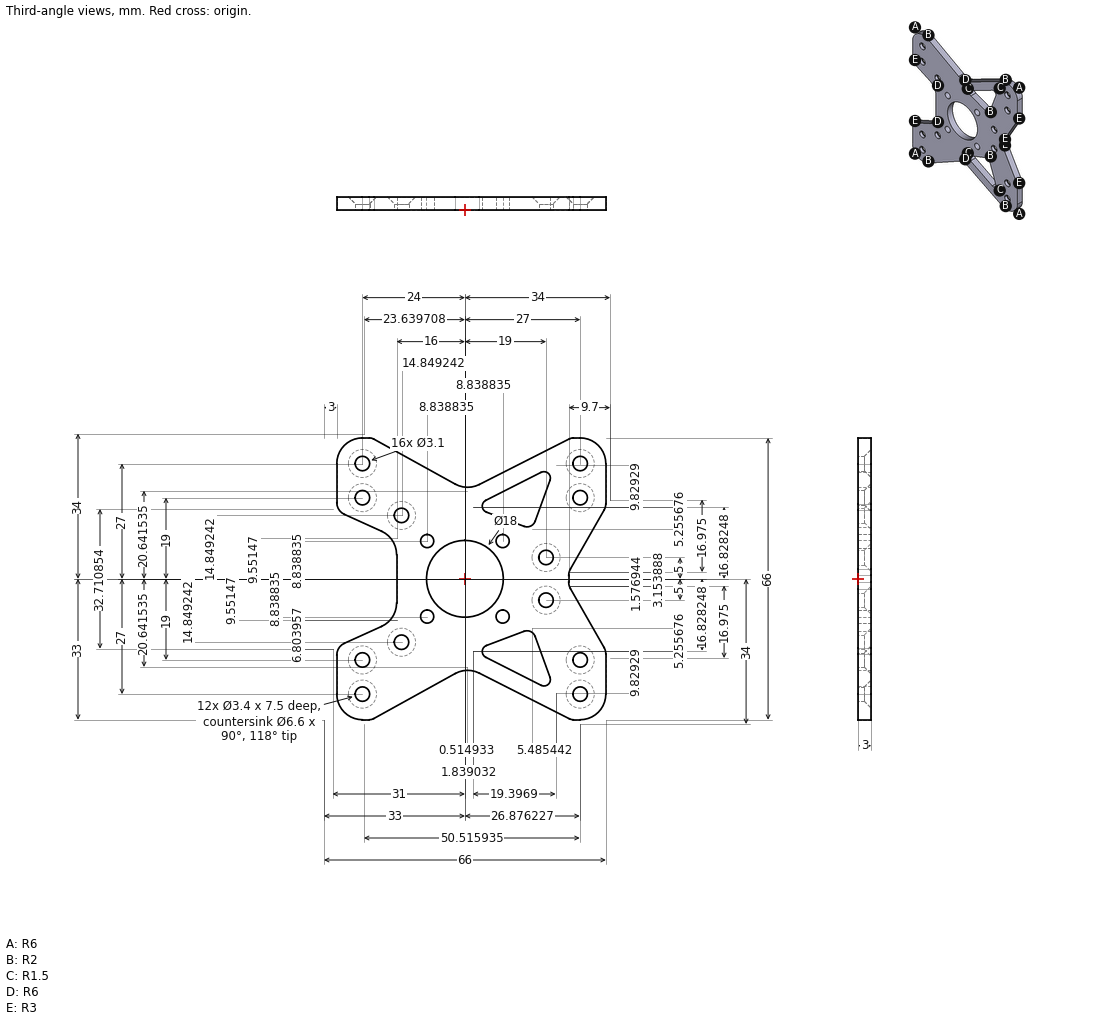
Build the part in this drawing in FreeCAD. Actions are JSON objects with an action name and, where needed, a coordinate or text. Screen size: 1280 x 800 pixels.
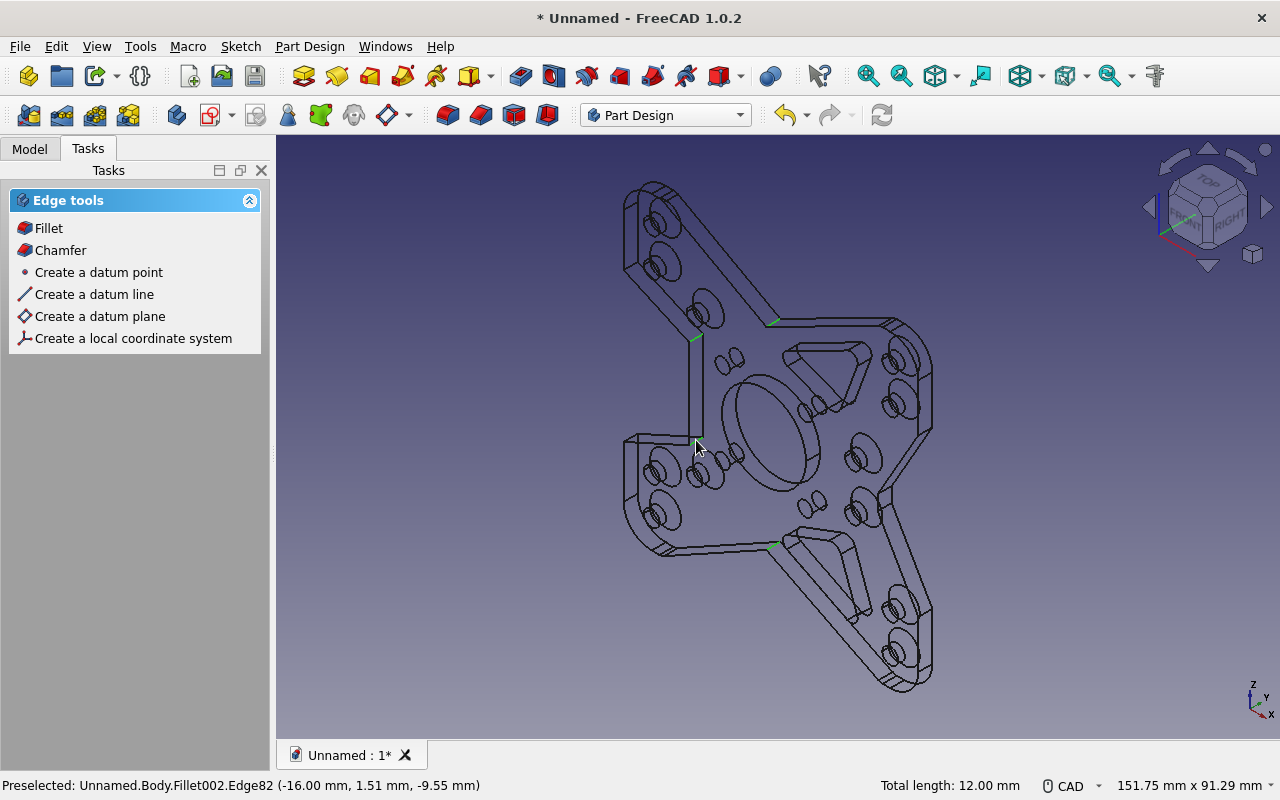
{"action": "key", "text": "v 1"}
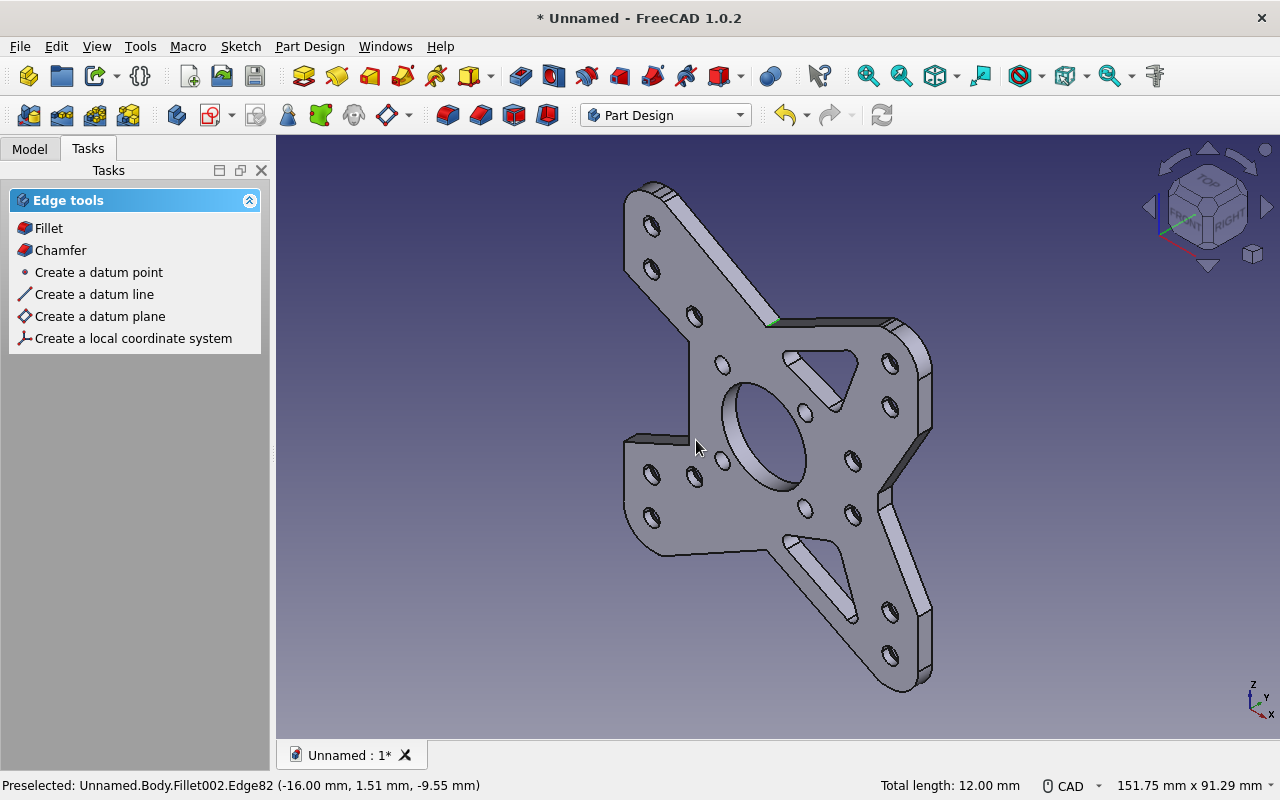
{"action": "left_click", "coordinate": [448, 116]}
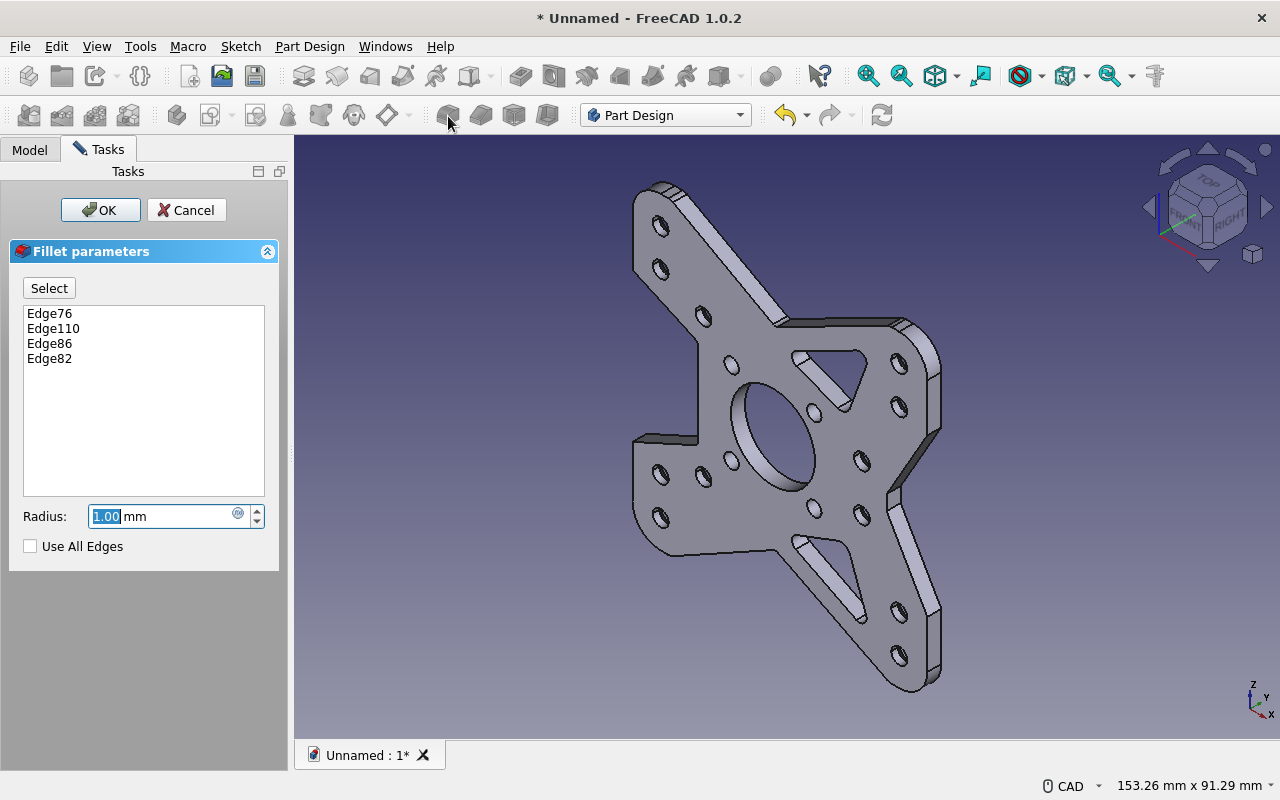
{"action": "type", "text": "6"}
{"action": "key", "text": "Tab"}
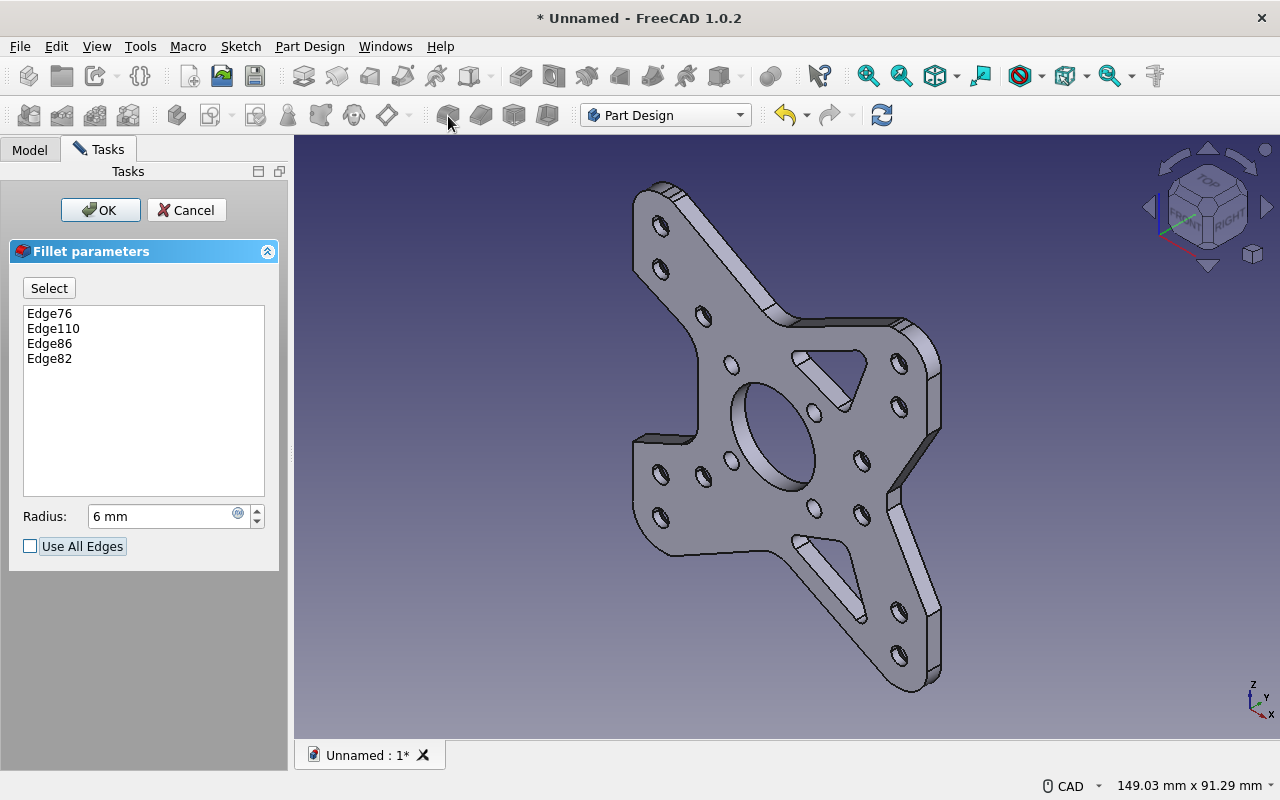
{"action": "left_click", "coordinate": [101, 210]}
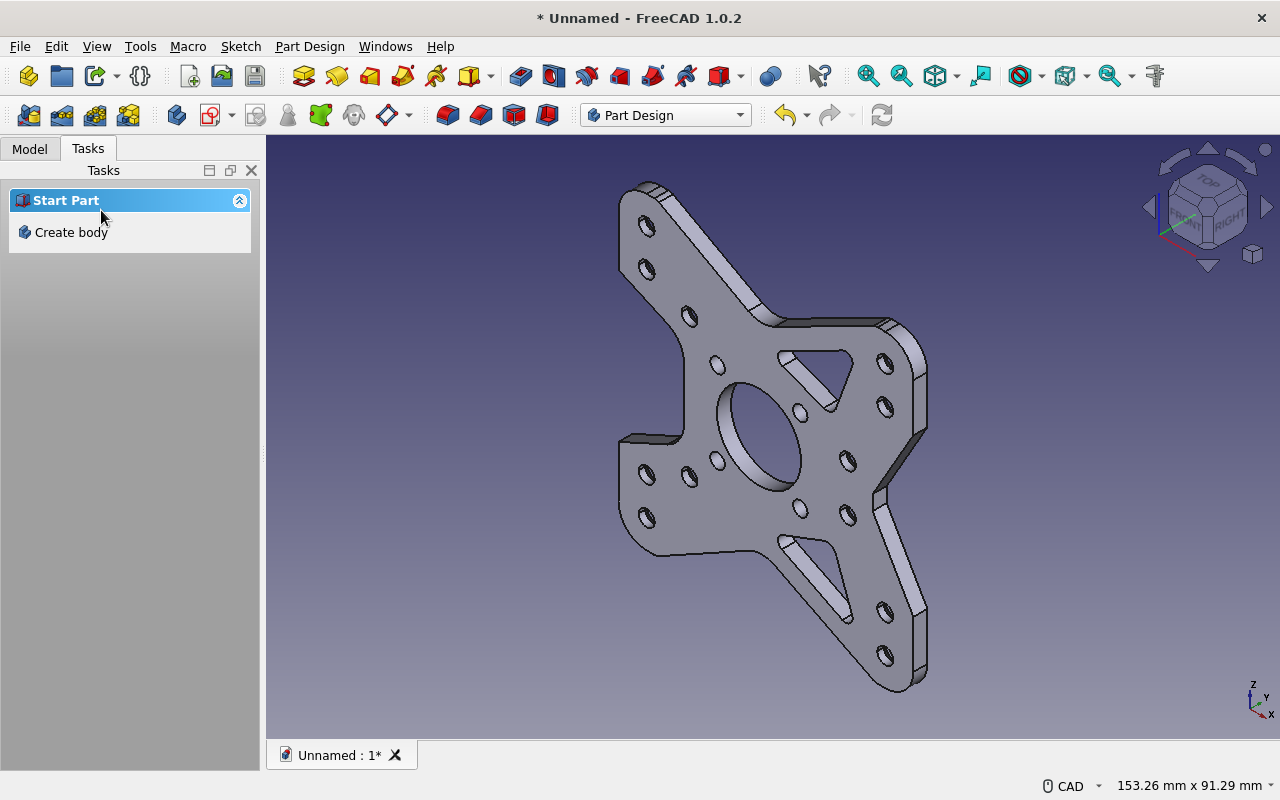
{"action": "scroll", "coordinate": [626, 437], "scroll_direction": "up", "scroll_amount": 4}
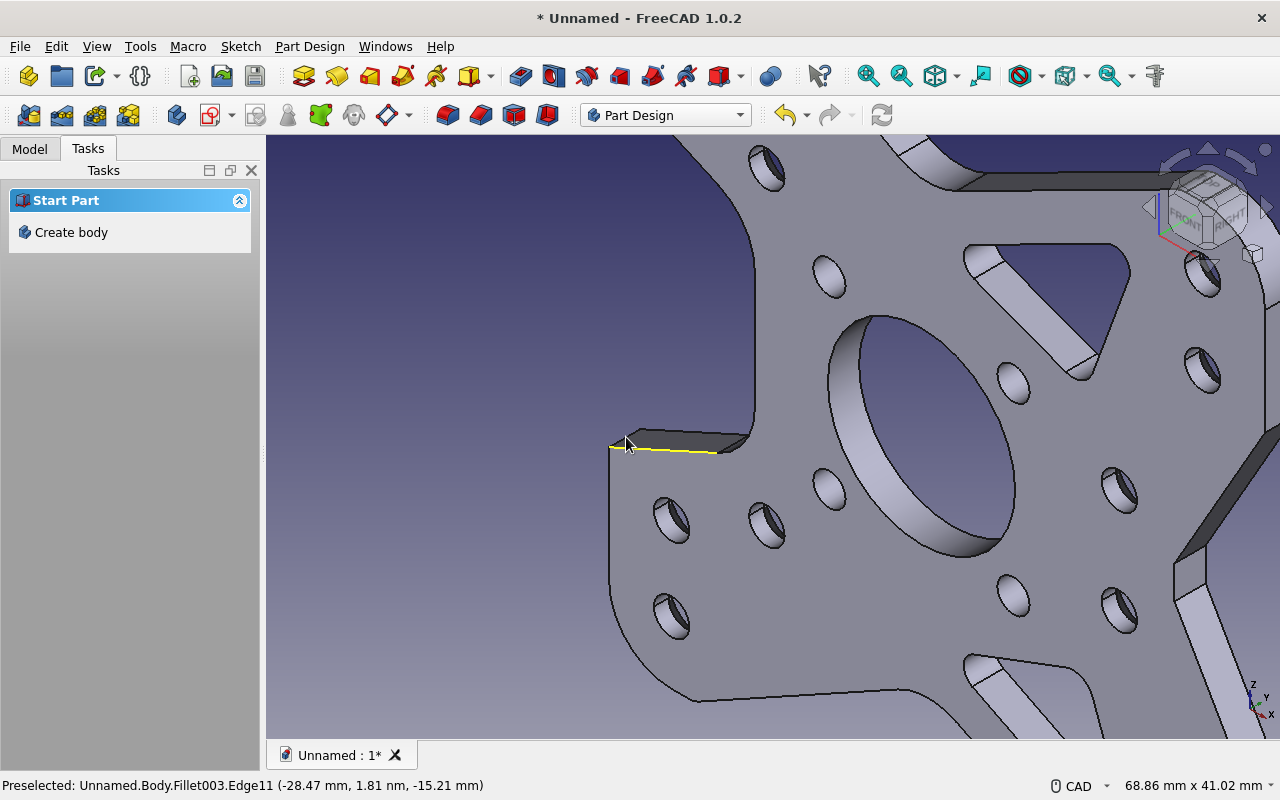
{"action": "left_click", "coordinate": [869, 76]}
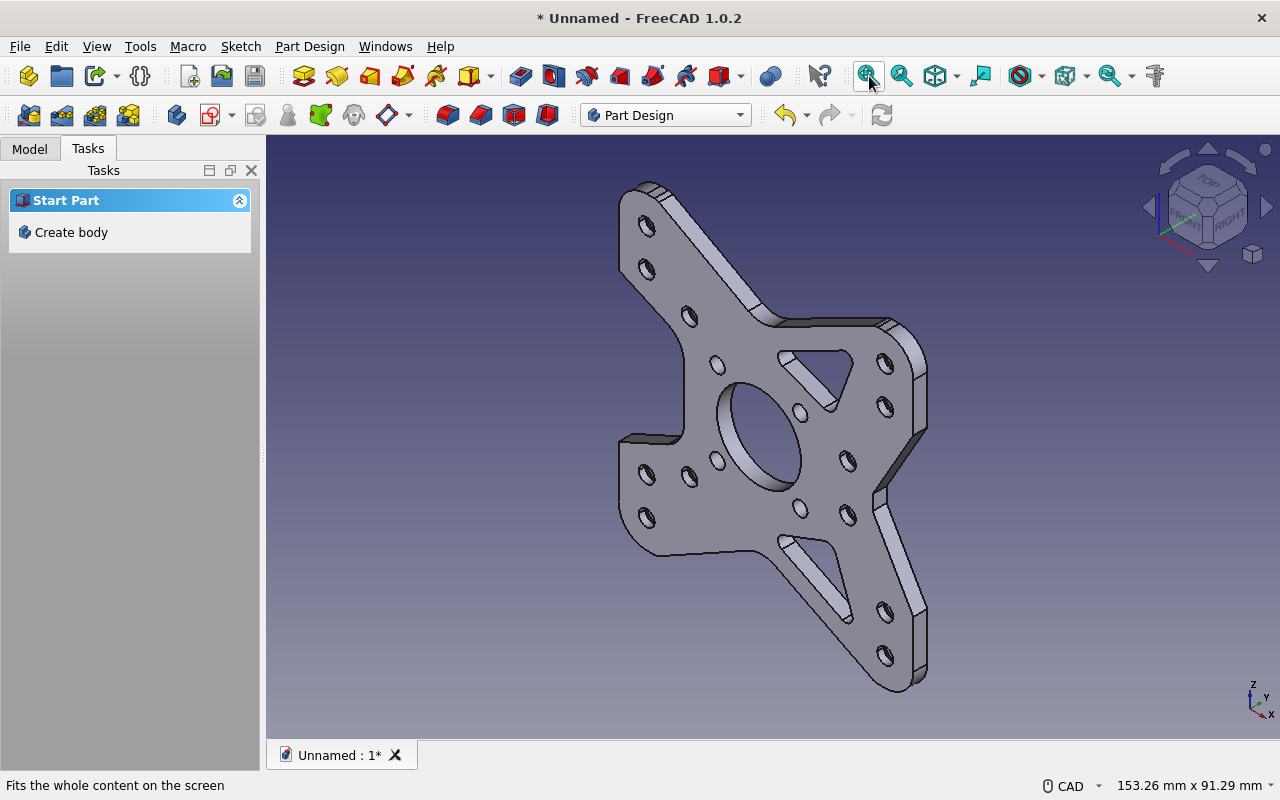
{"action": "key", "text": "2"}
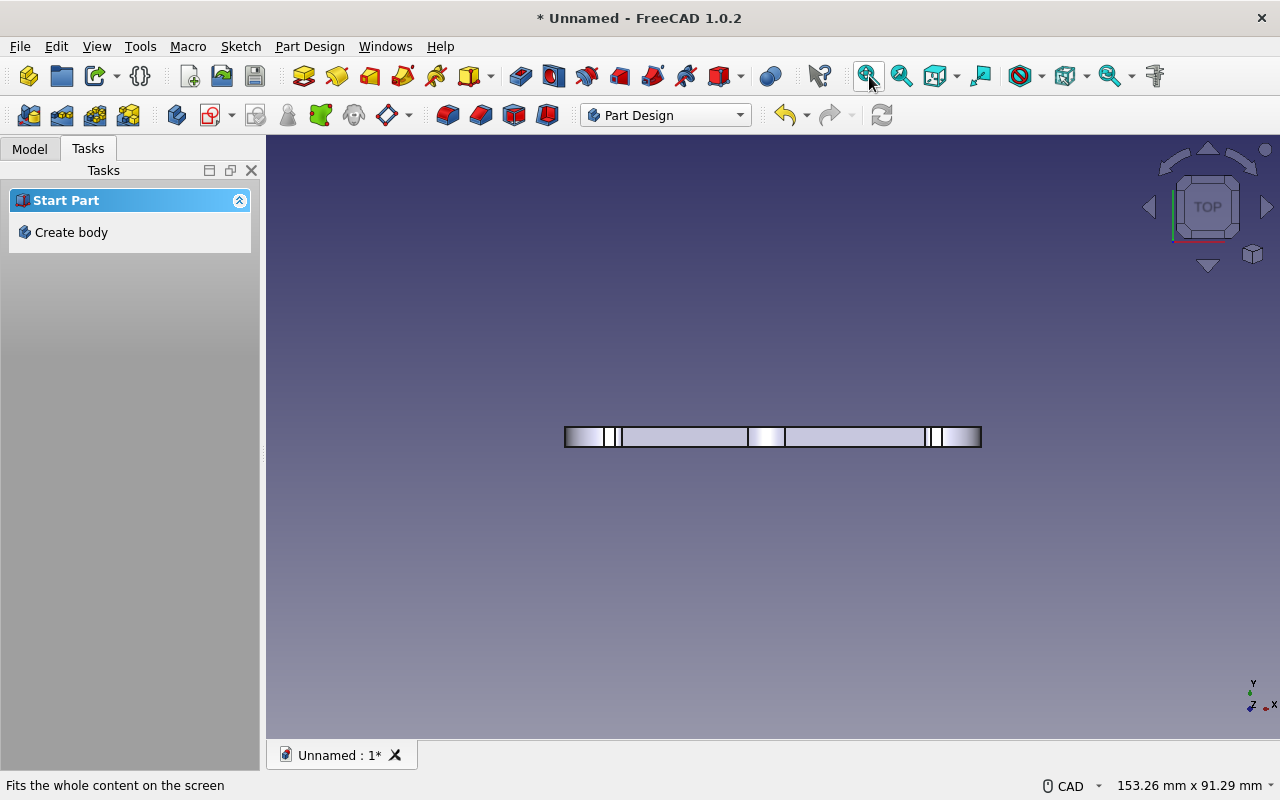
{"action": "left_click", "coordinate": [869, 76]}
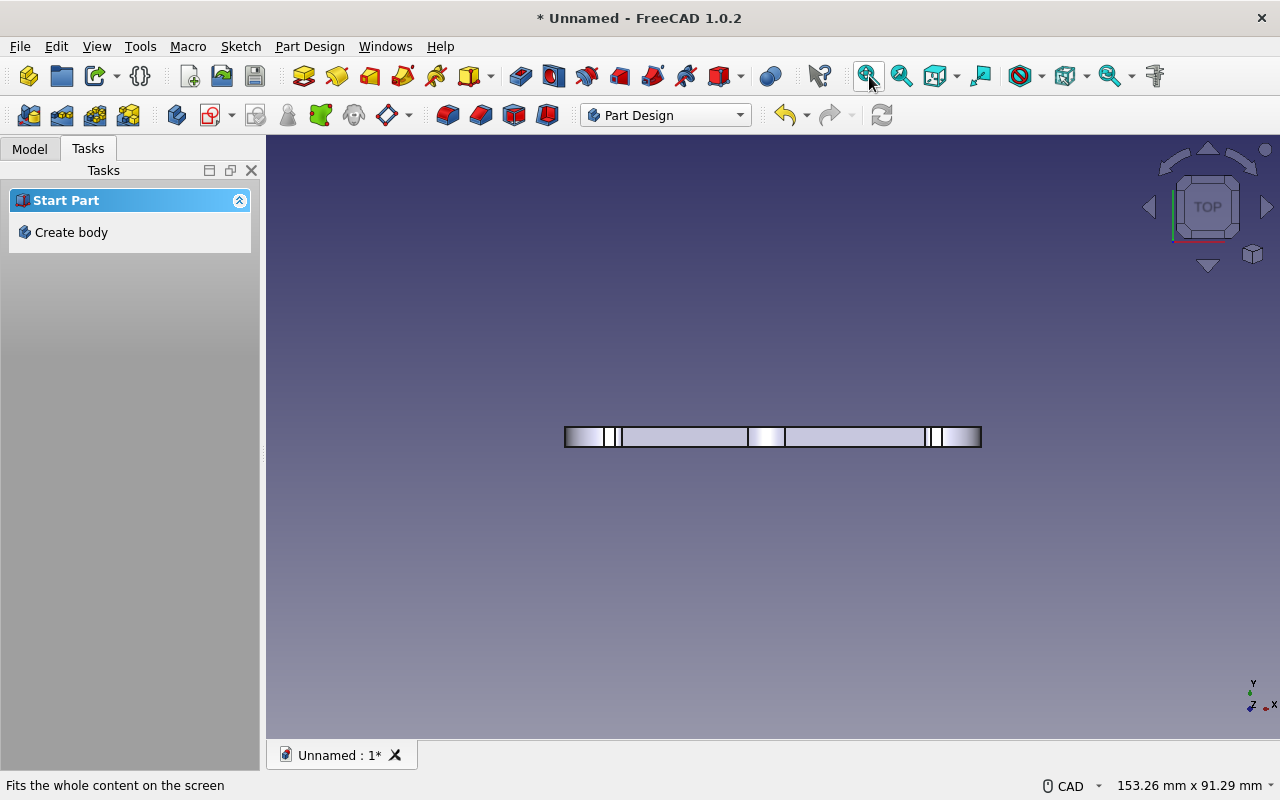
{"action": "scroll", "coordinate": [565, 436], "scroll_direction": "up", "scroll_amount": 4}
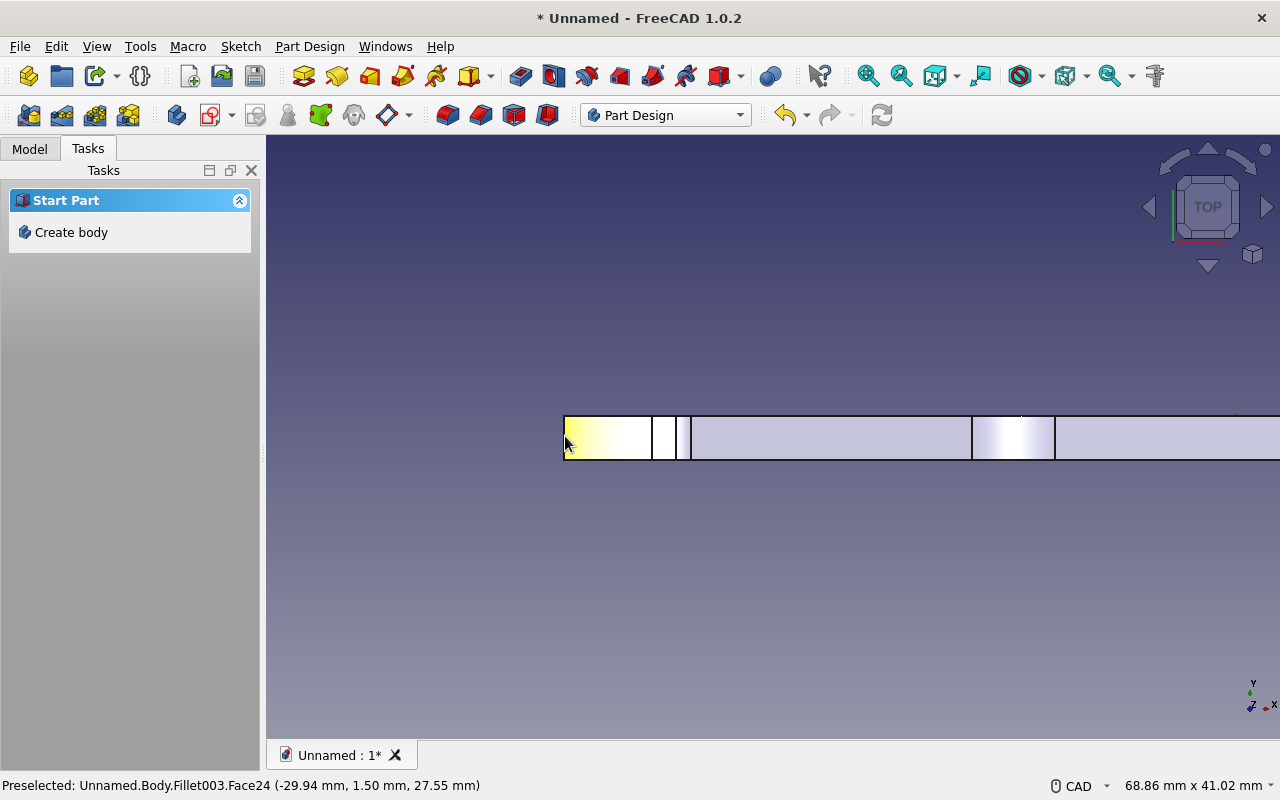
{"action": "left_click", "coordinate": [869, 76]}